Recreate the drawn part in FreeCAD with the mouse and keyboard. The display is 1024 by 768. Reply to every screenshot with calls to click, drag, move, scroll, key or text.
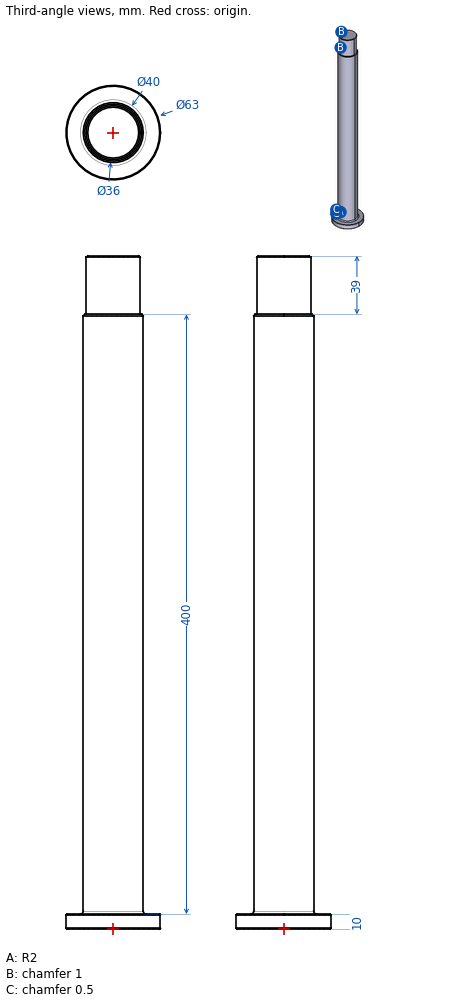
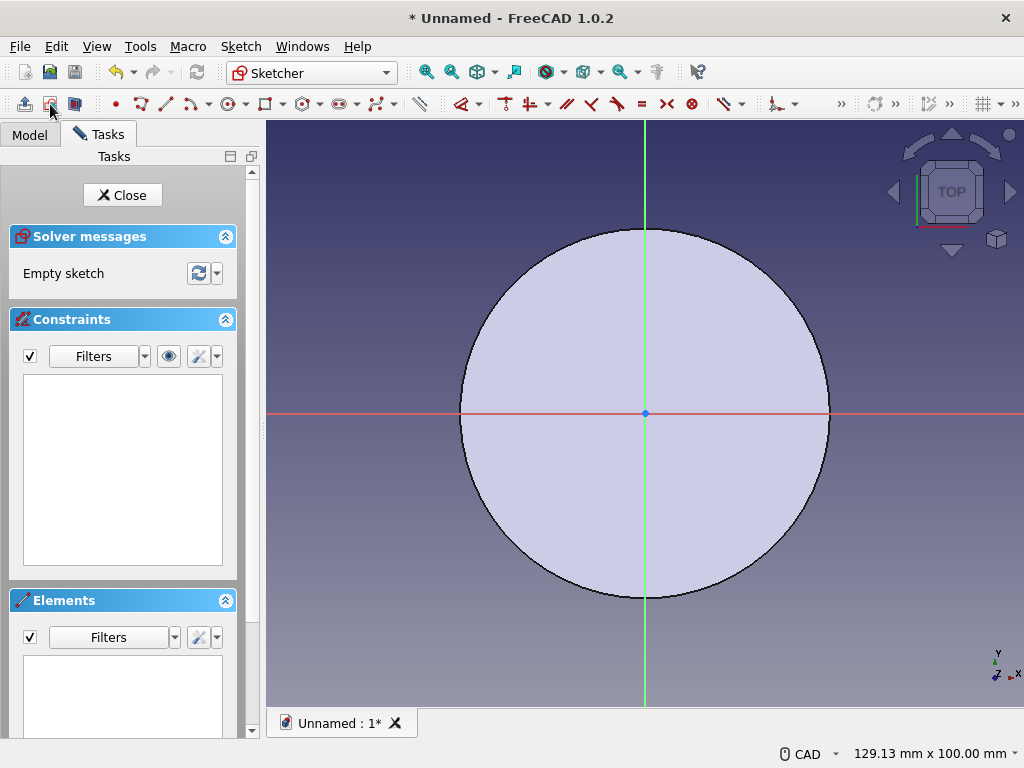
scroll(784, 413, up, 2)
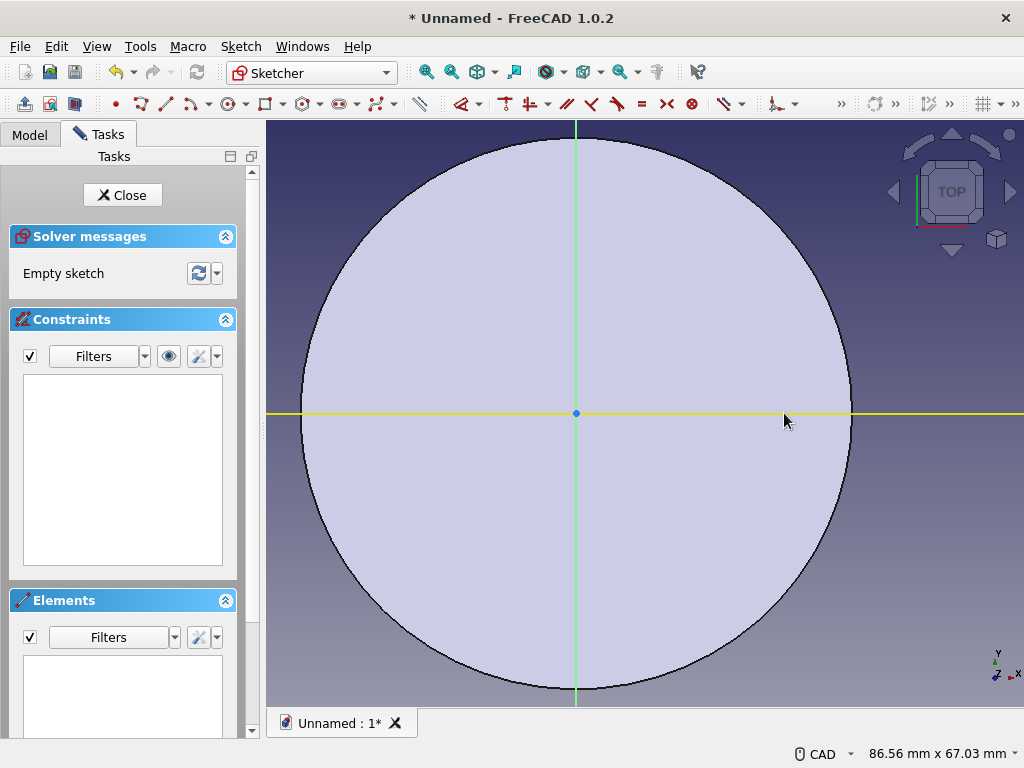
click(228, 104)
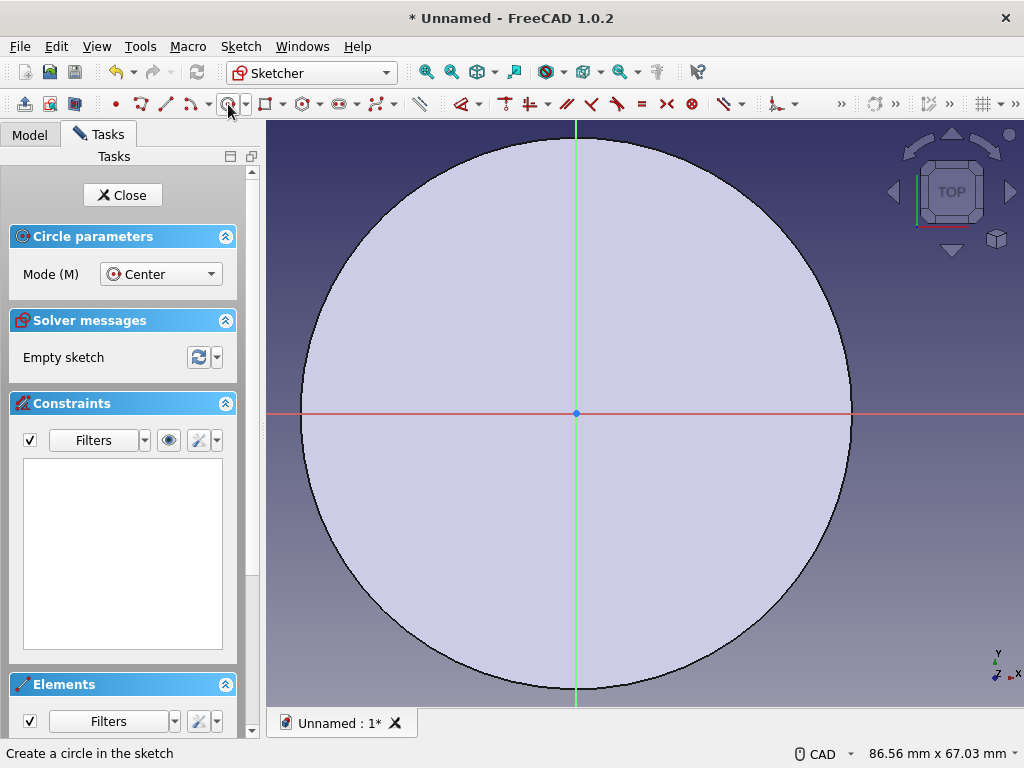
click(576, 414)
move(700, 290)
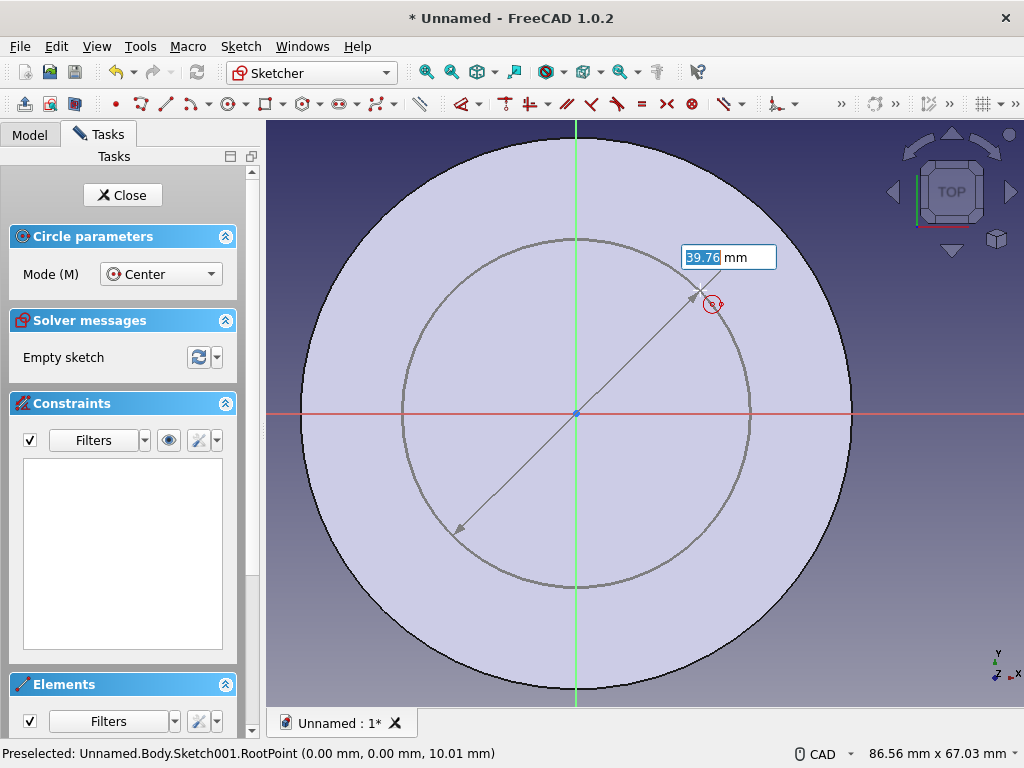
text(40)
key(Return)
key(Escape)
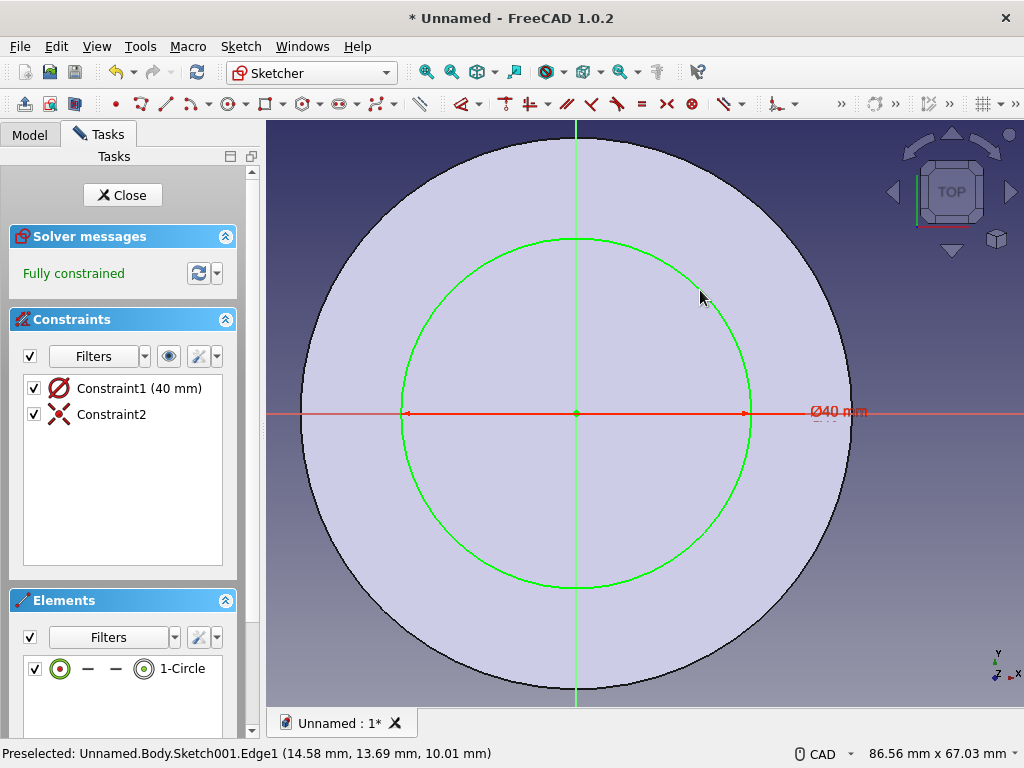
click(123, 195)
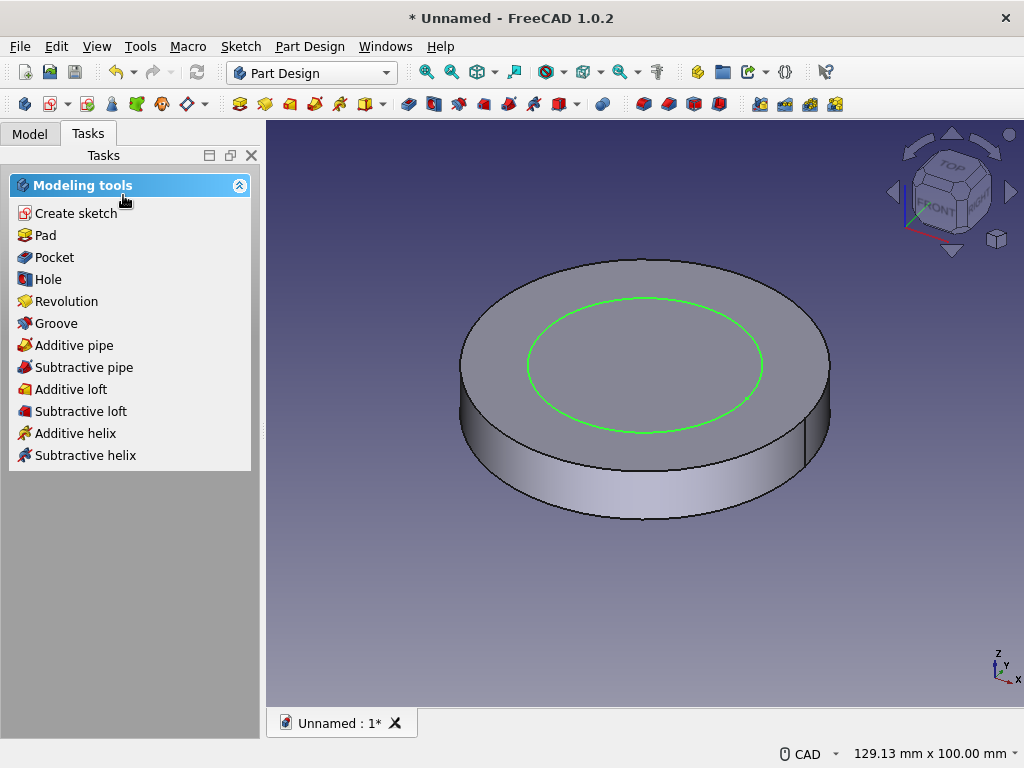
click(240, 104)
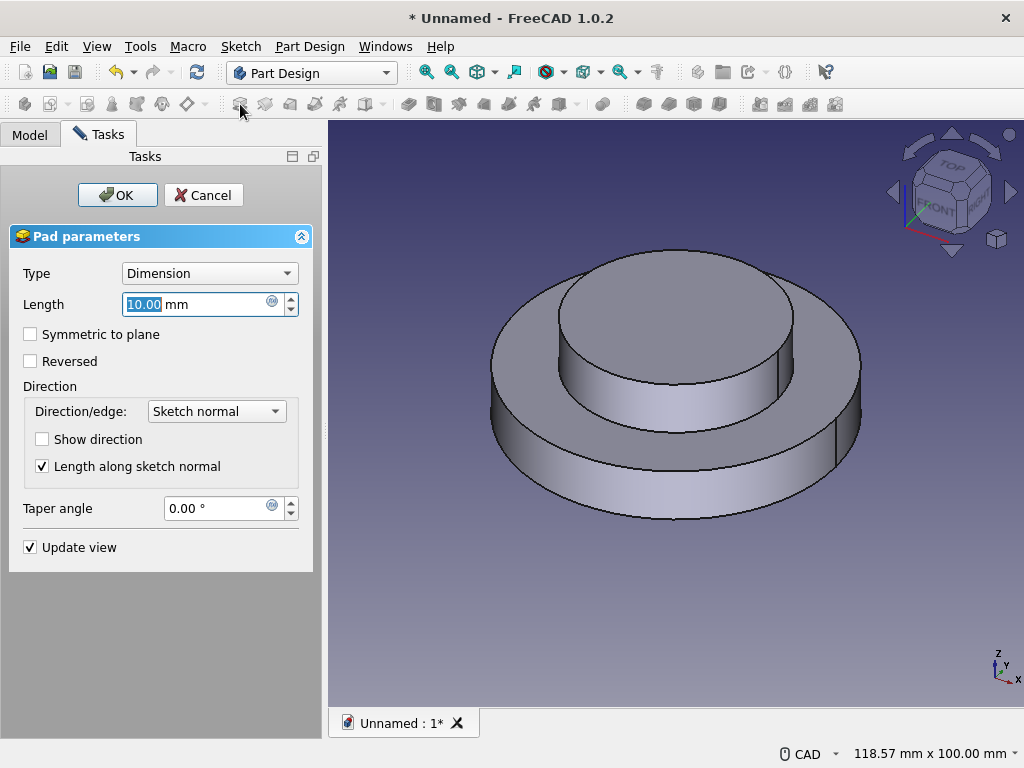
text(400)
key(Tab)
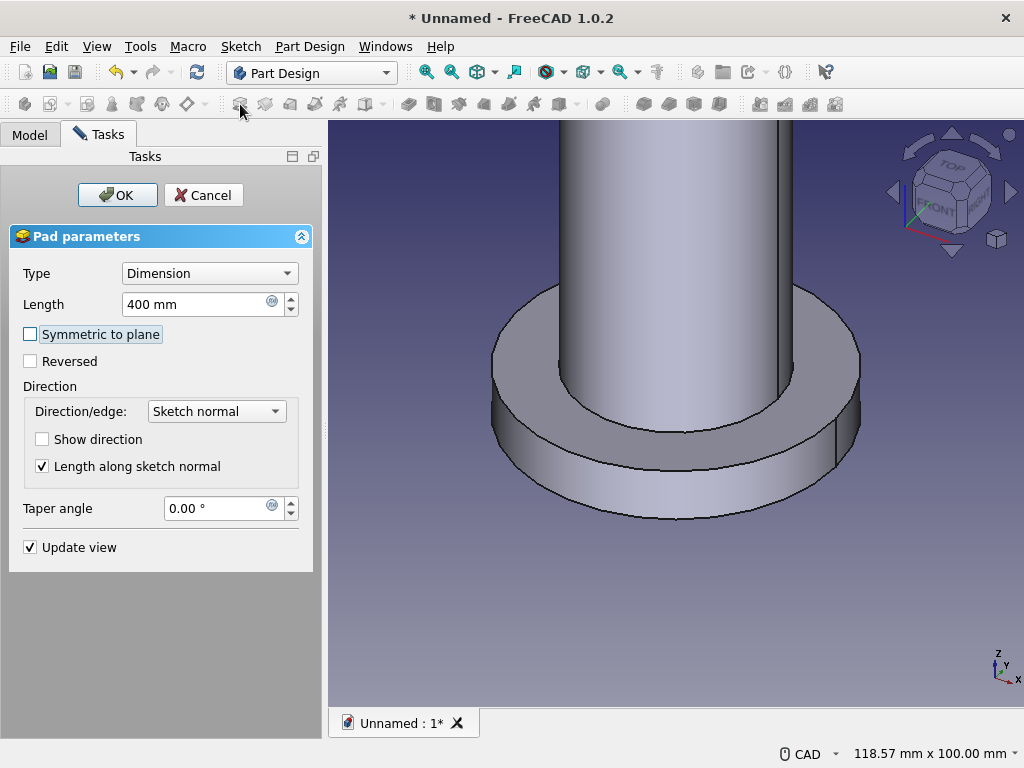
click(118, 195)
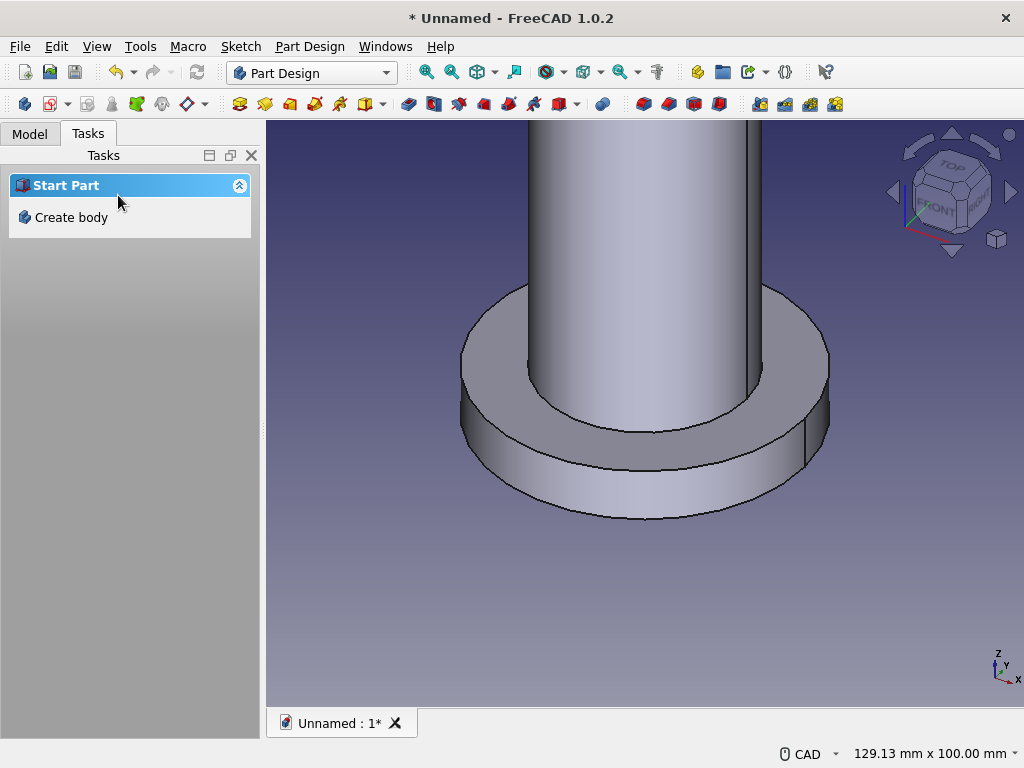
click(427, 72)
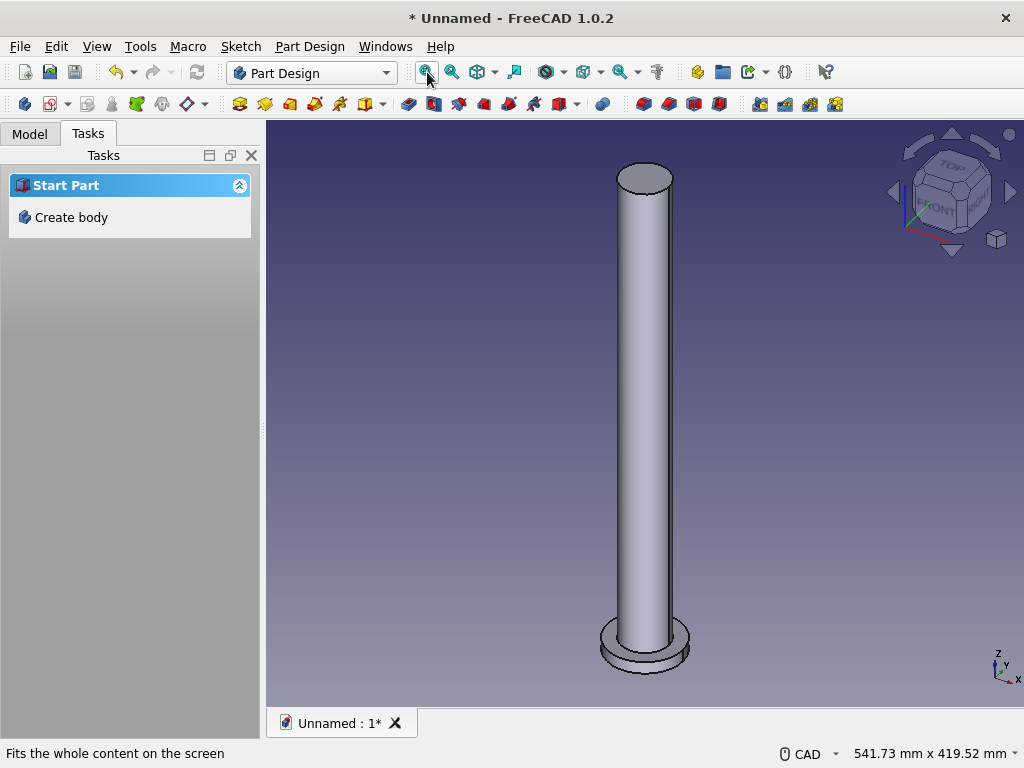
click(645, 178)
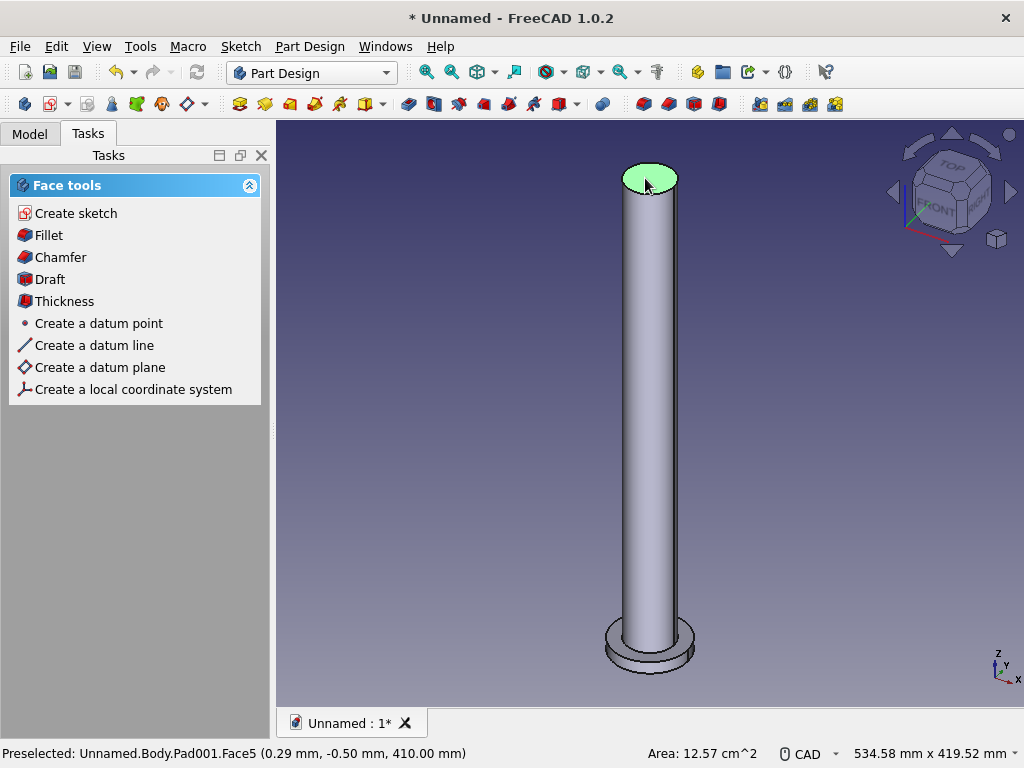
click(50, 104)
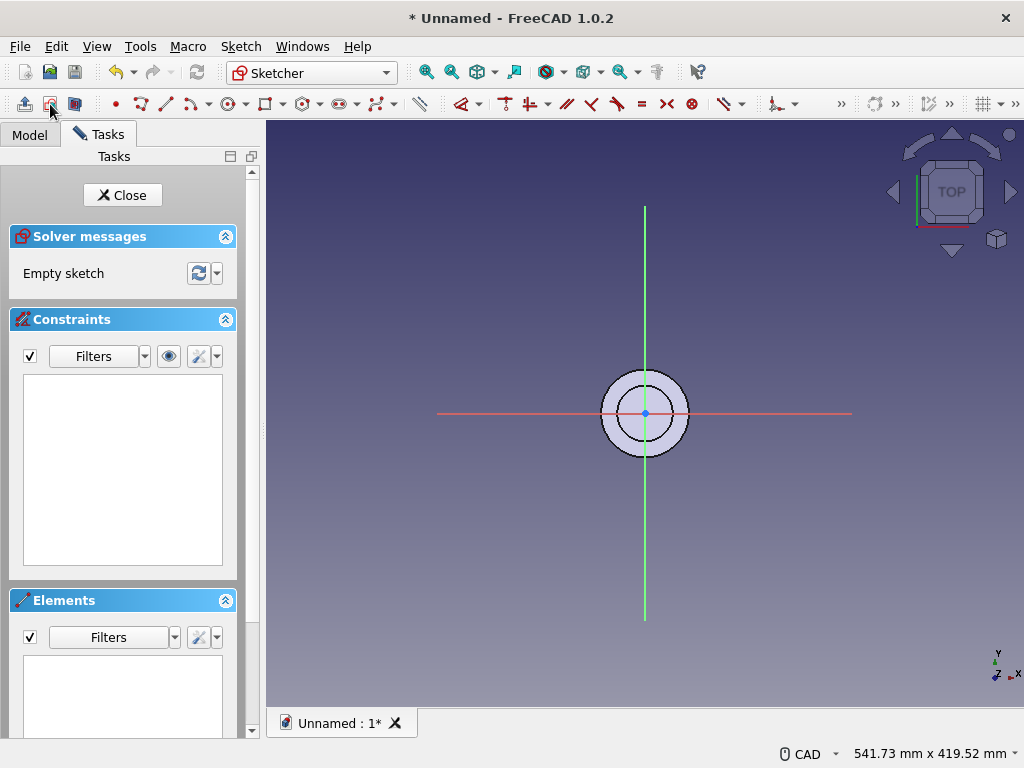
scroll(656, 414, up, 10)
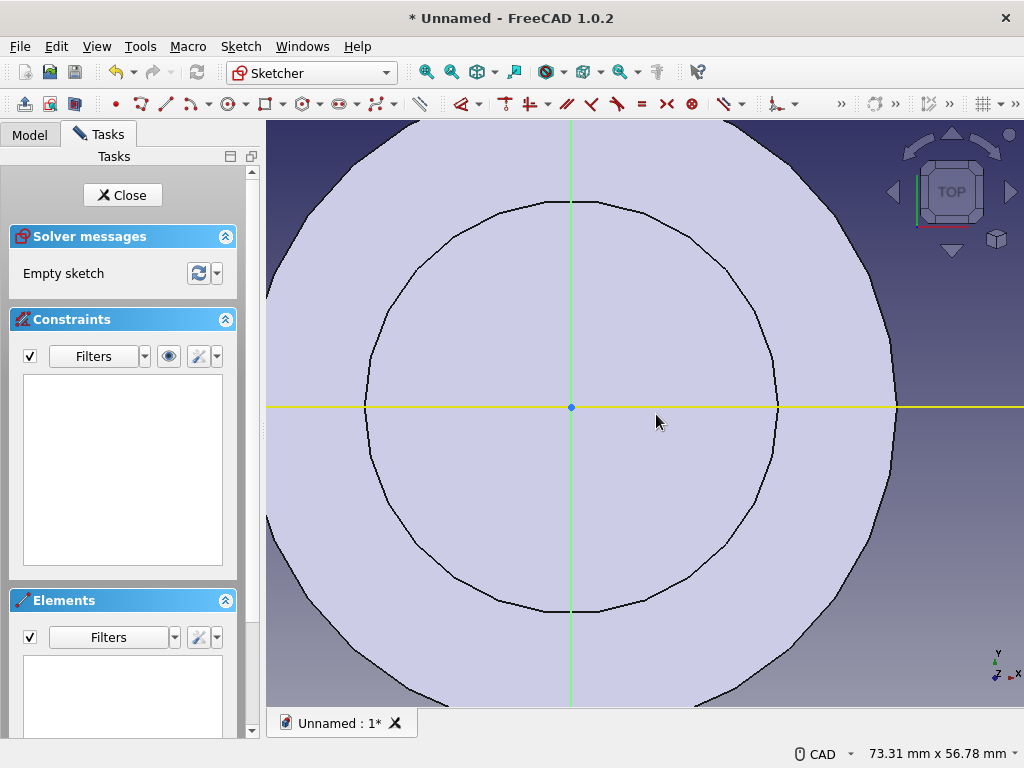
click(228, 104)